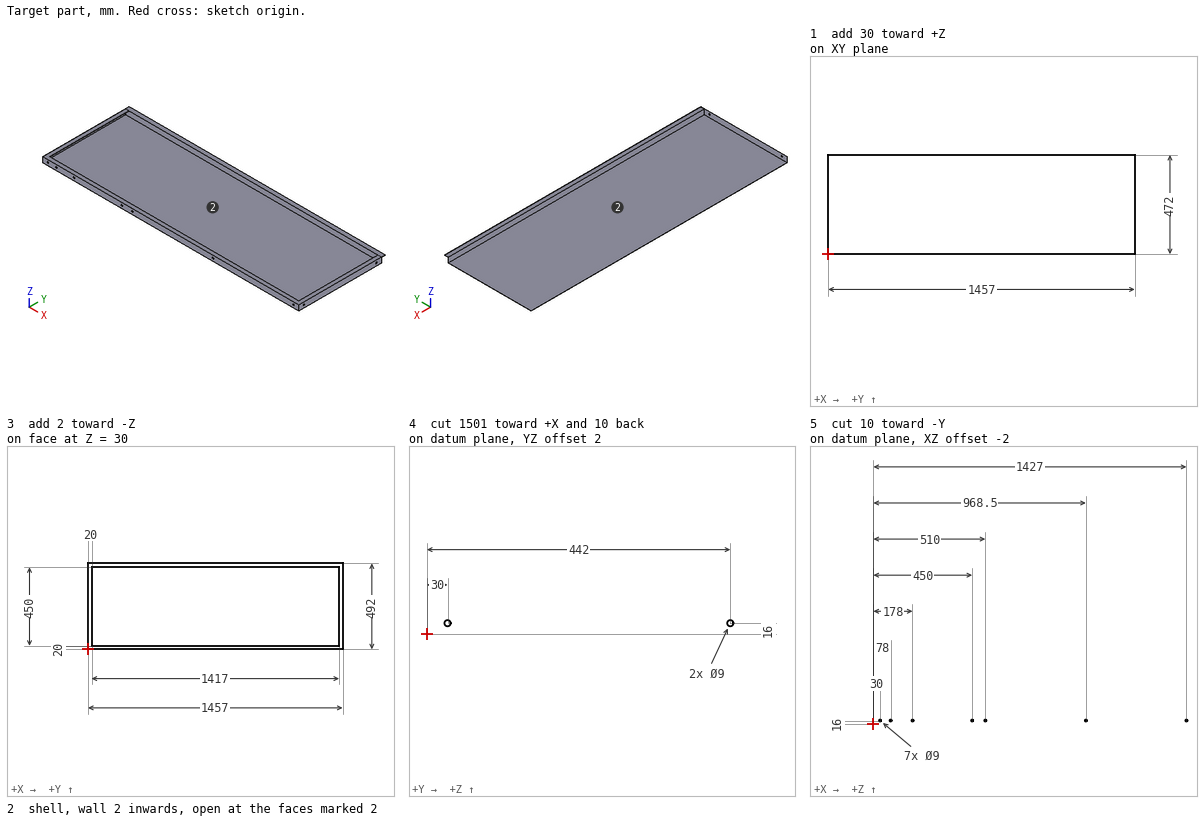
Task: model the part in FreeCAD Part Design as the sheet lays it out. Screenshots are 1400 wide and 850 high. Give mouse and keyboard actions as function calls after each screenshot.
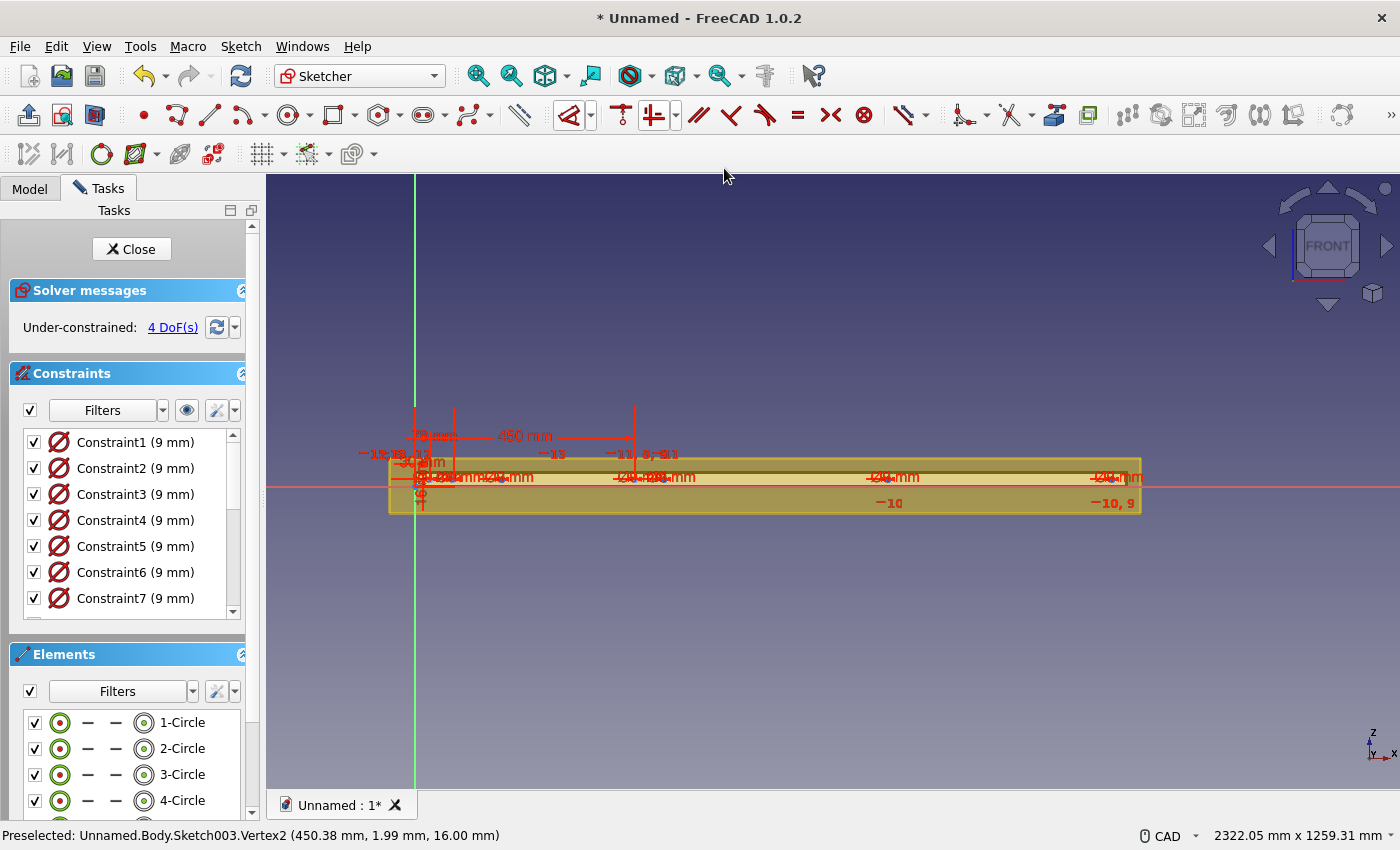
click(664, 479)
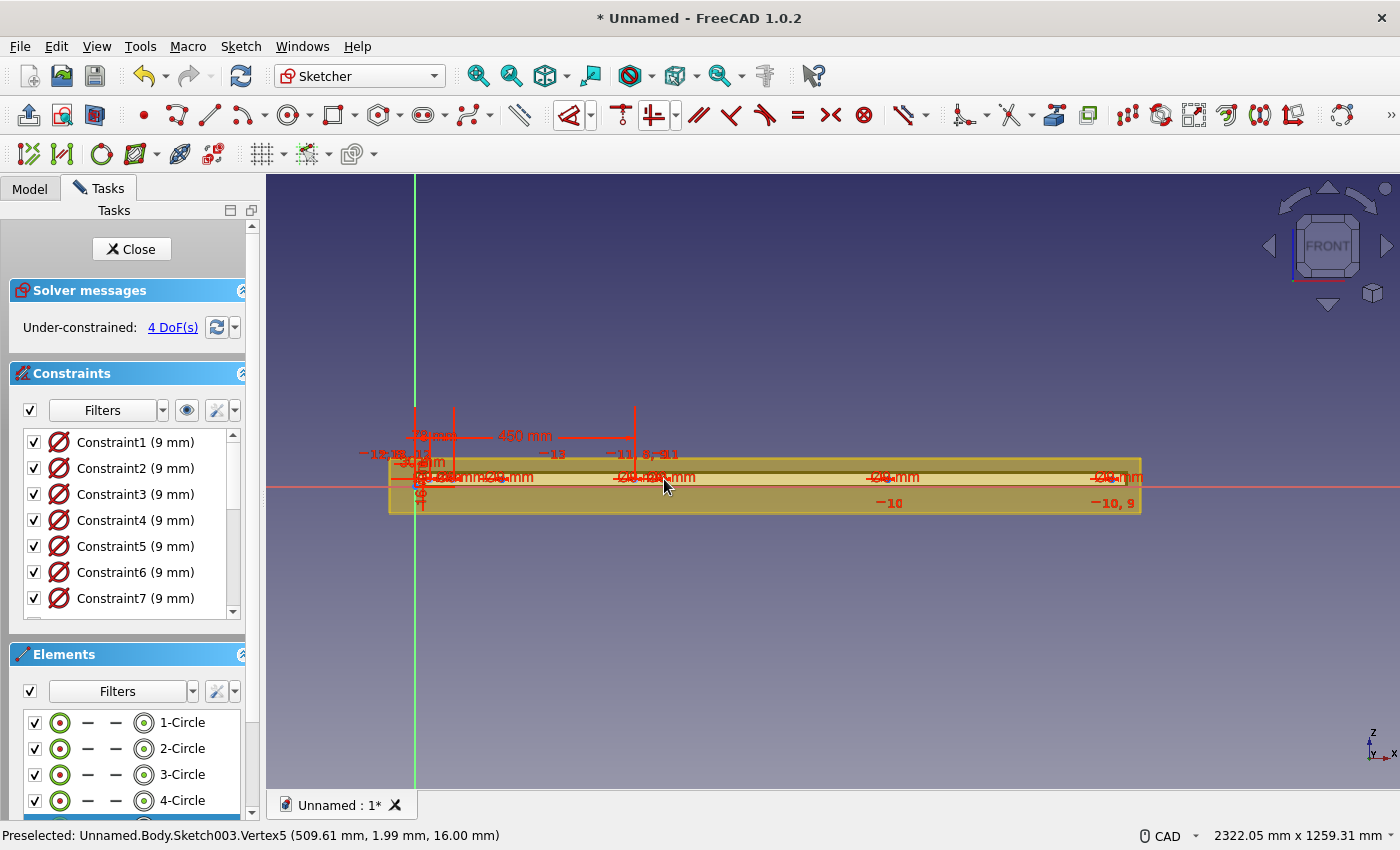
key(l)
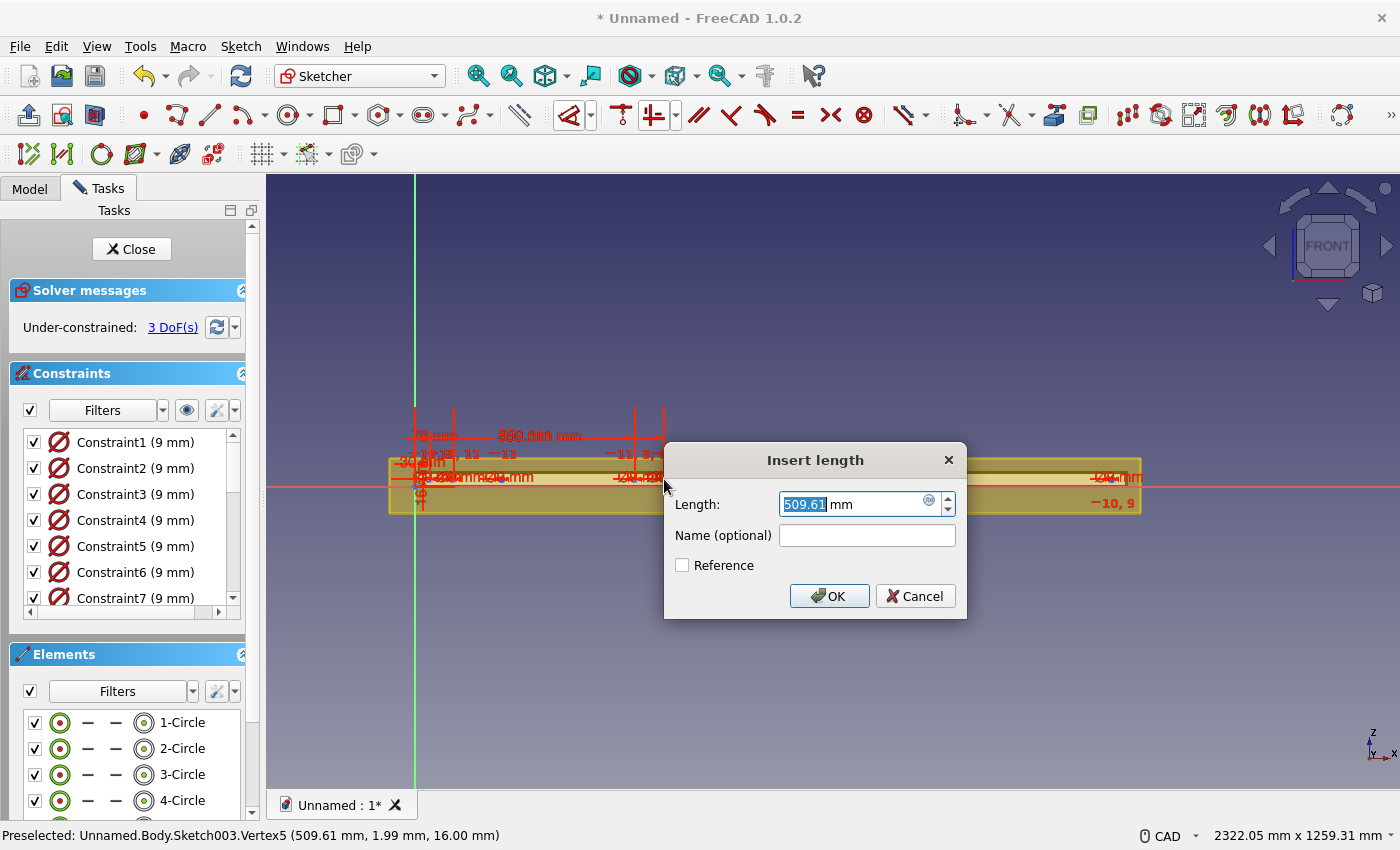
text(510)
key(Return)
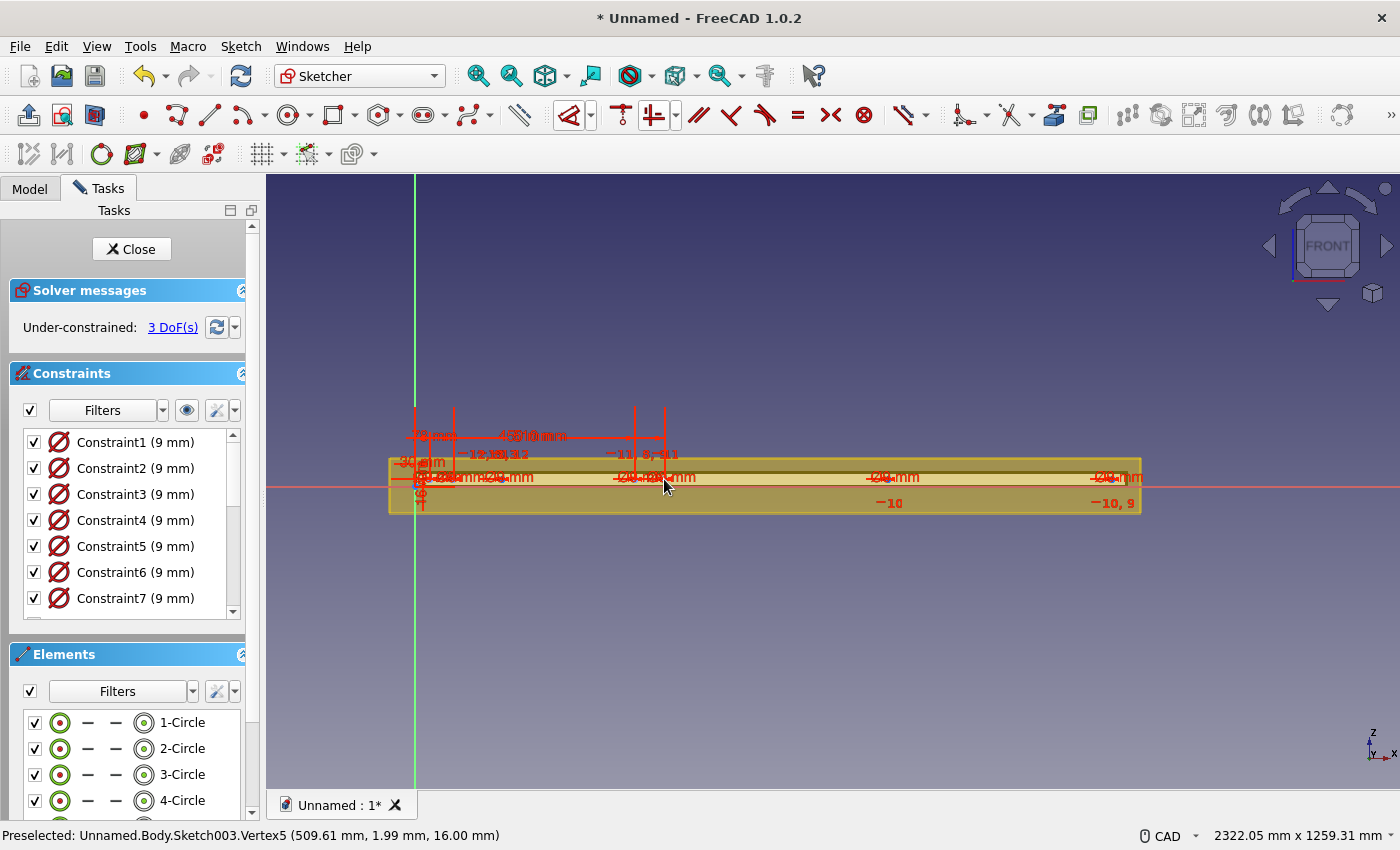
click(502, 479)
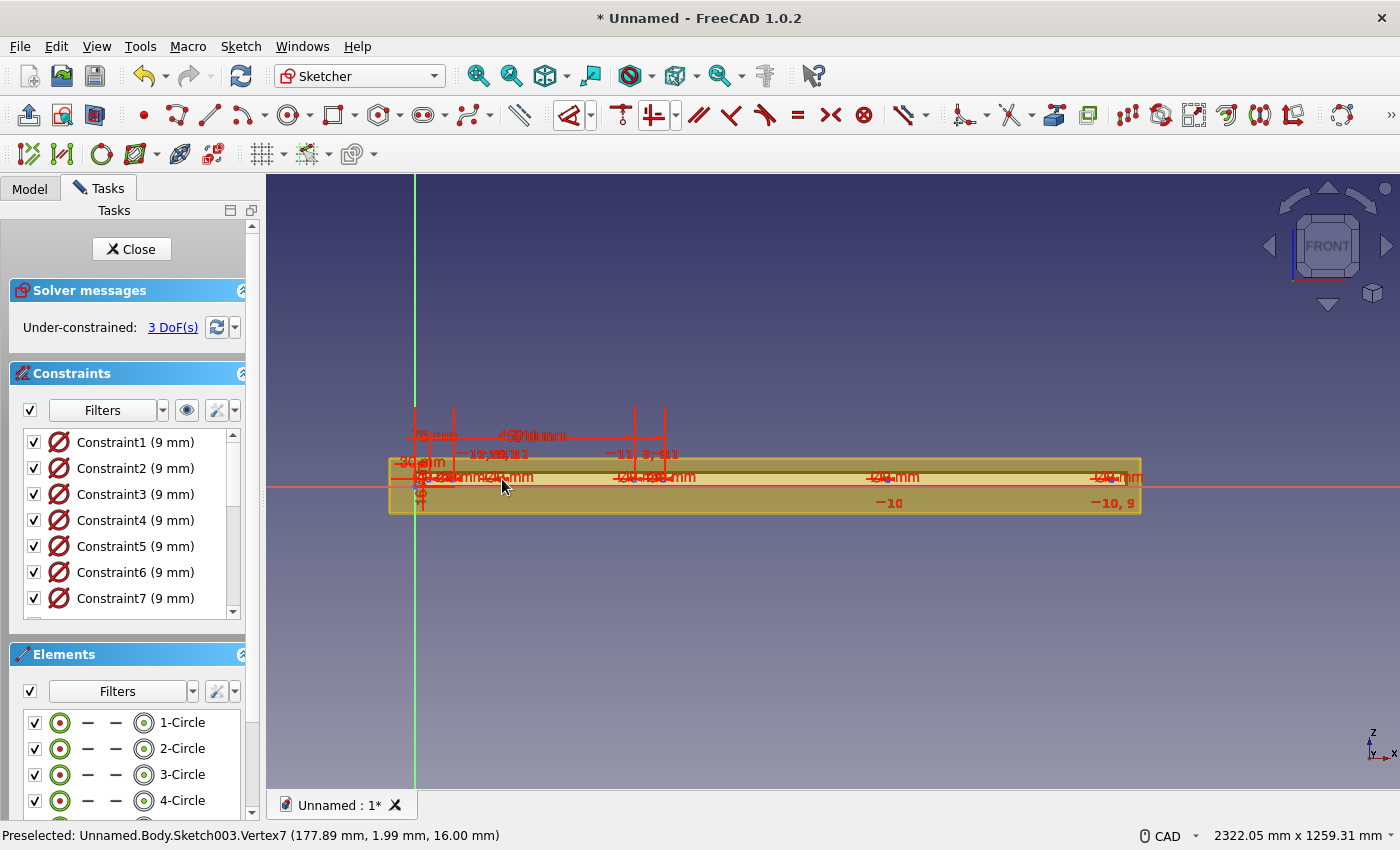
key(l)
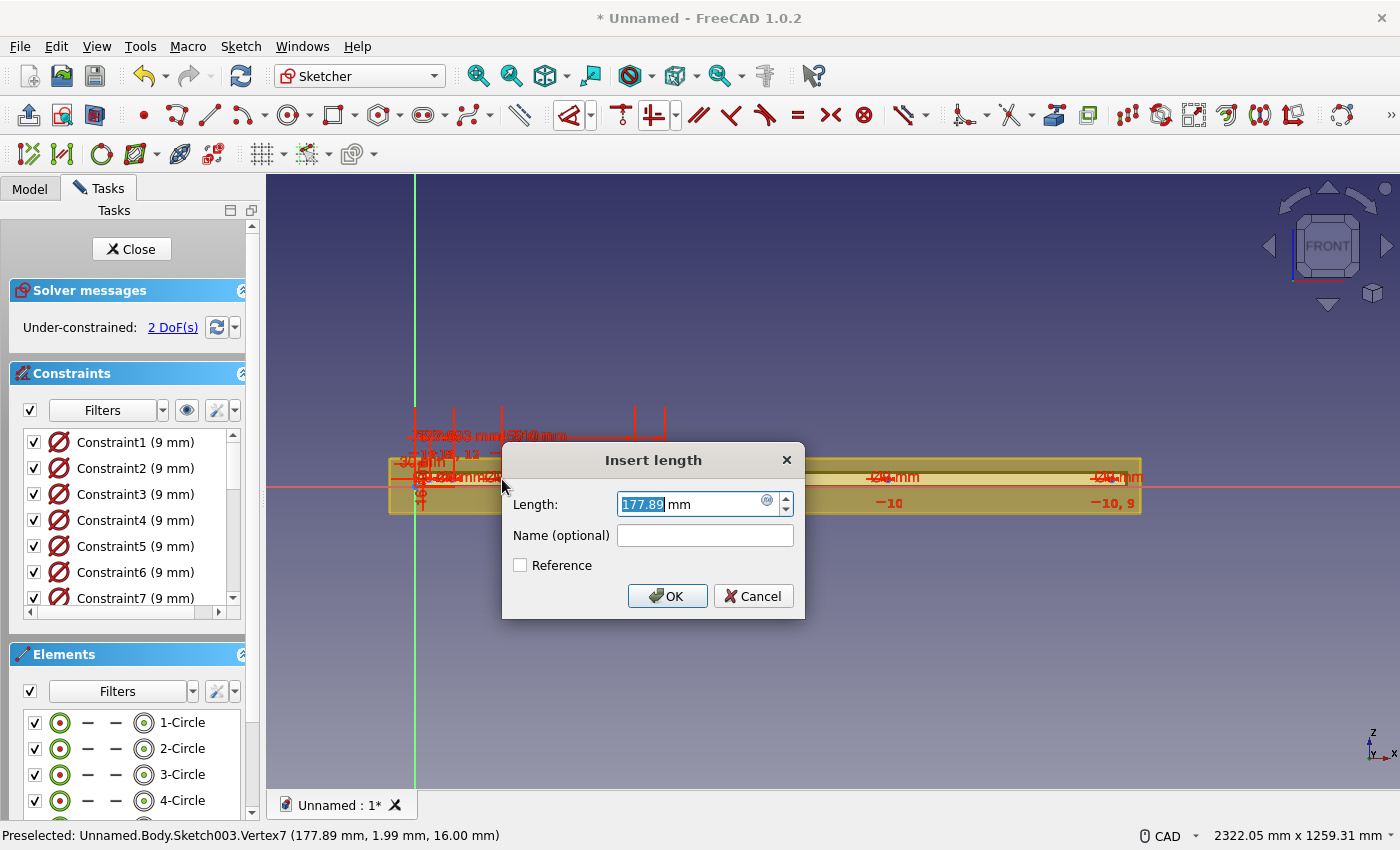
text(178)
key(Return)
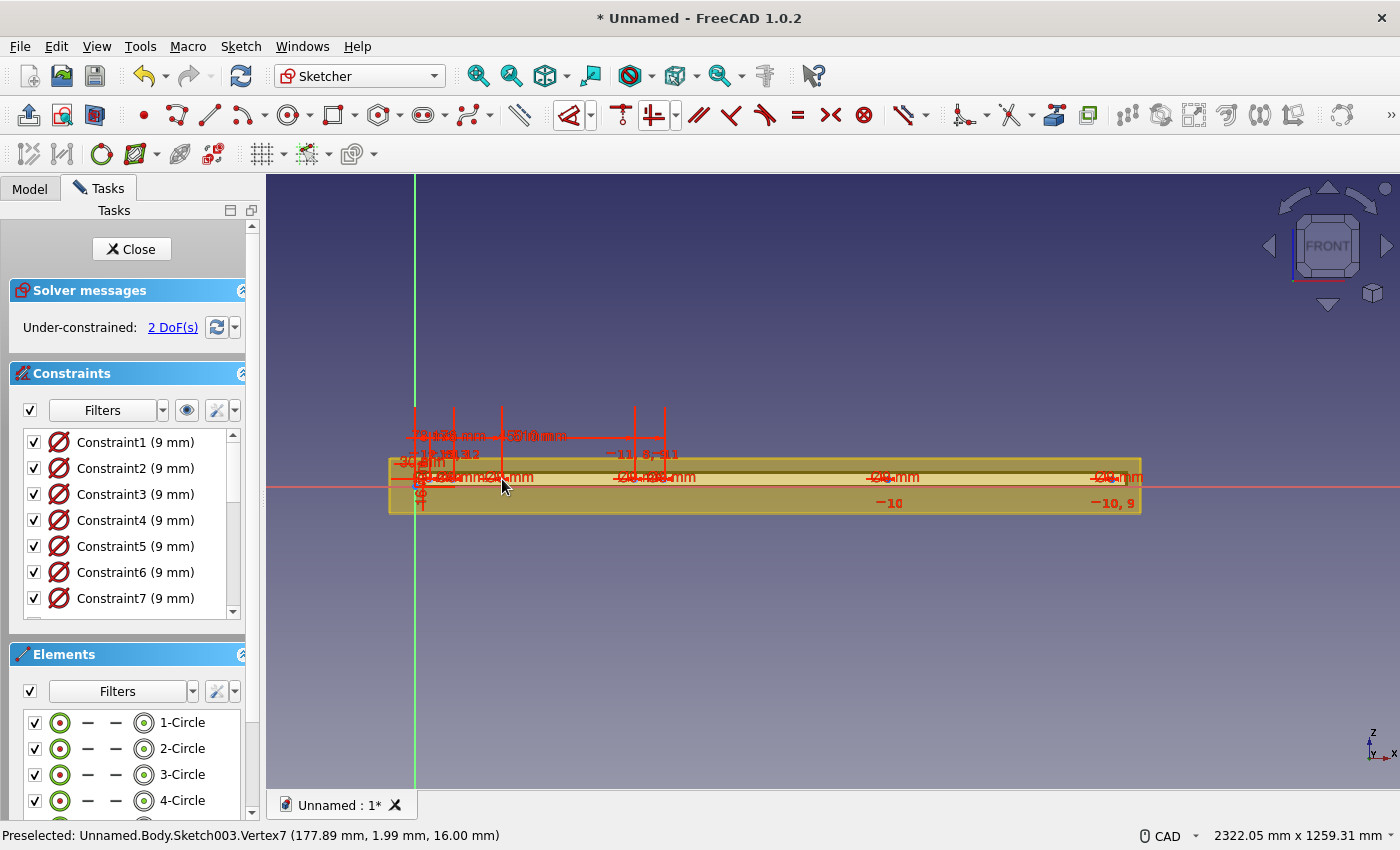
click(1112, 479)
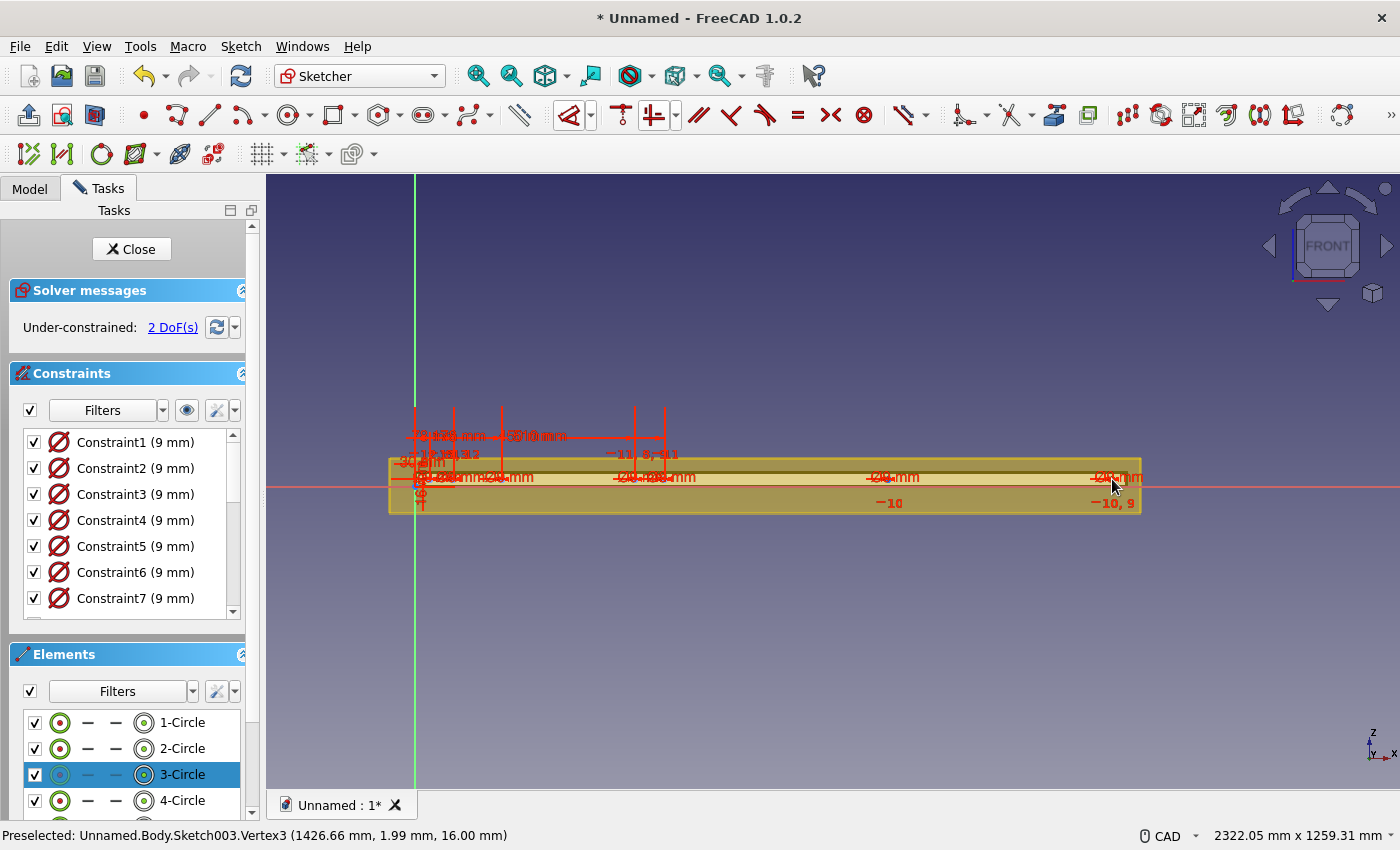
key(l)